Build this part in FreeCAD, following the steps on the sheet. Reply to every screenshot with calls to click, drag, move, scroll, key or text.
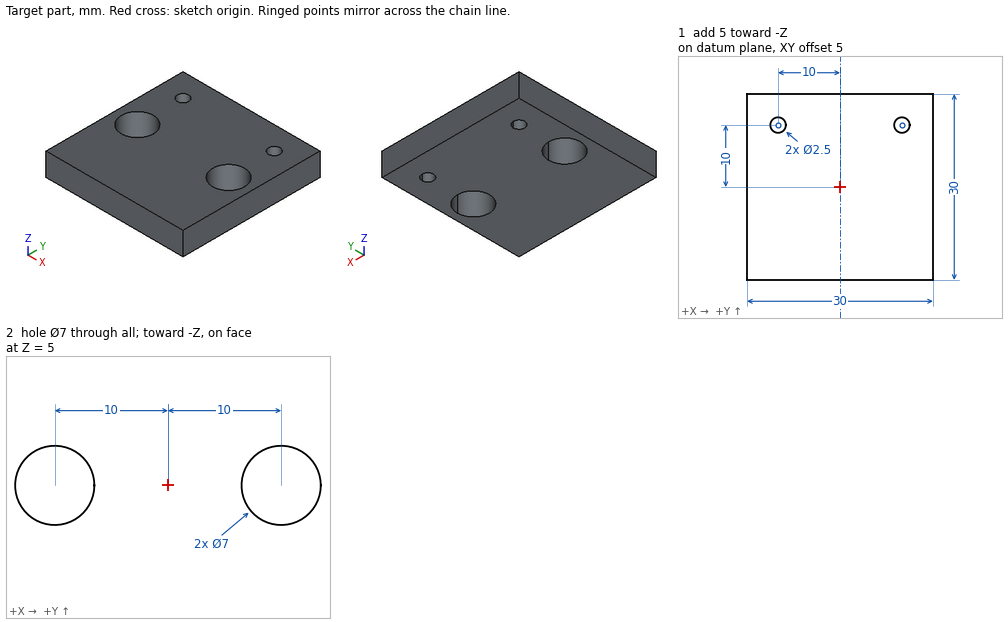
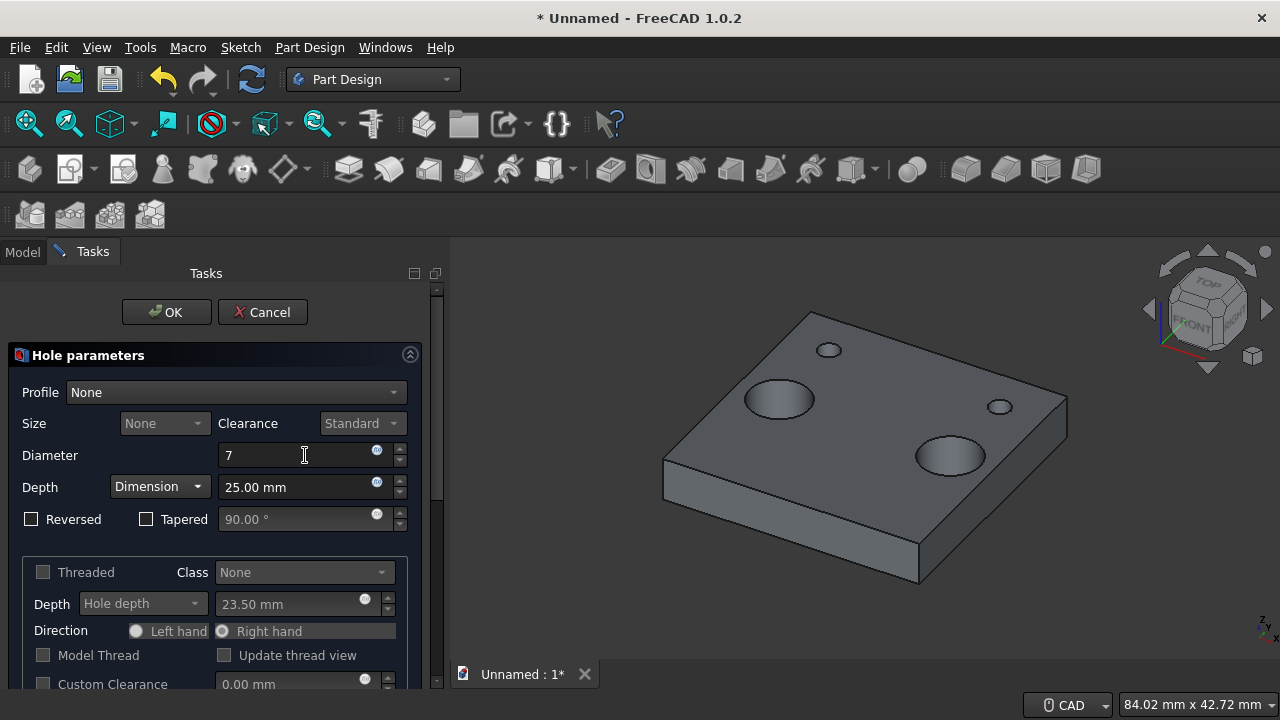
click(161, 486)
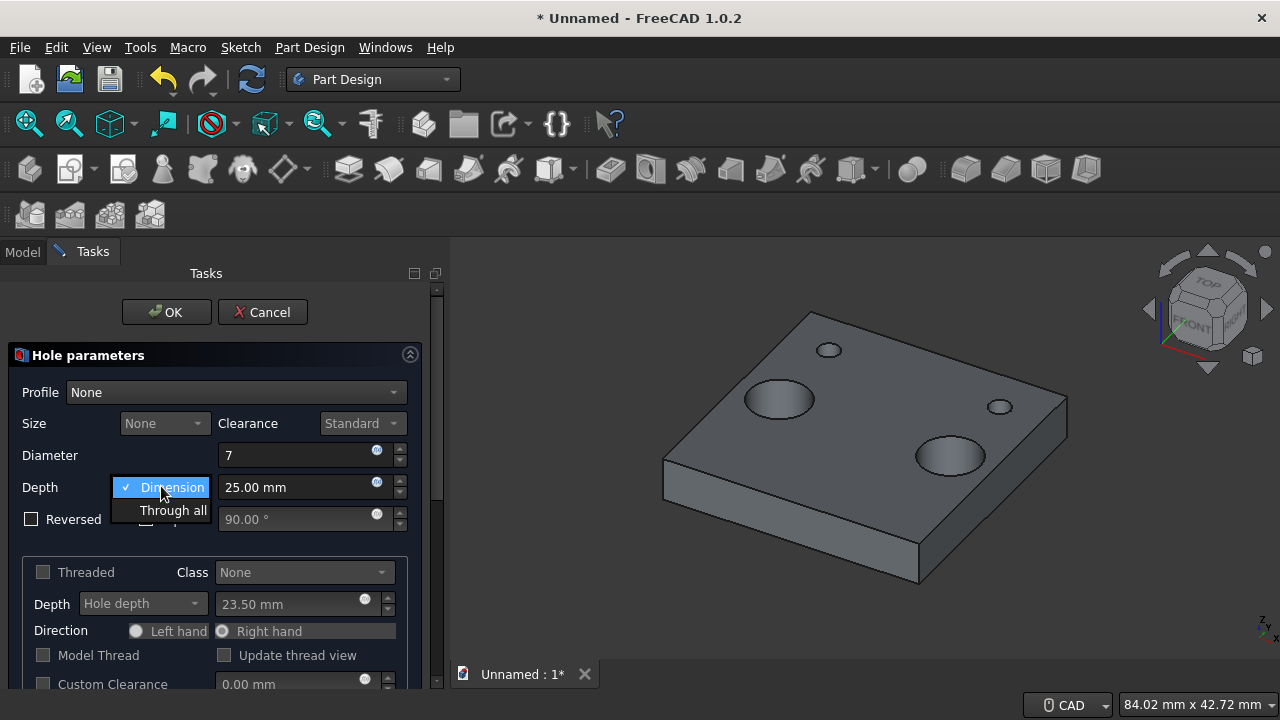
click(160, 510)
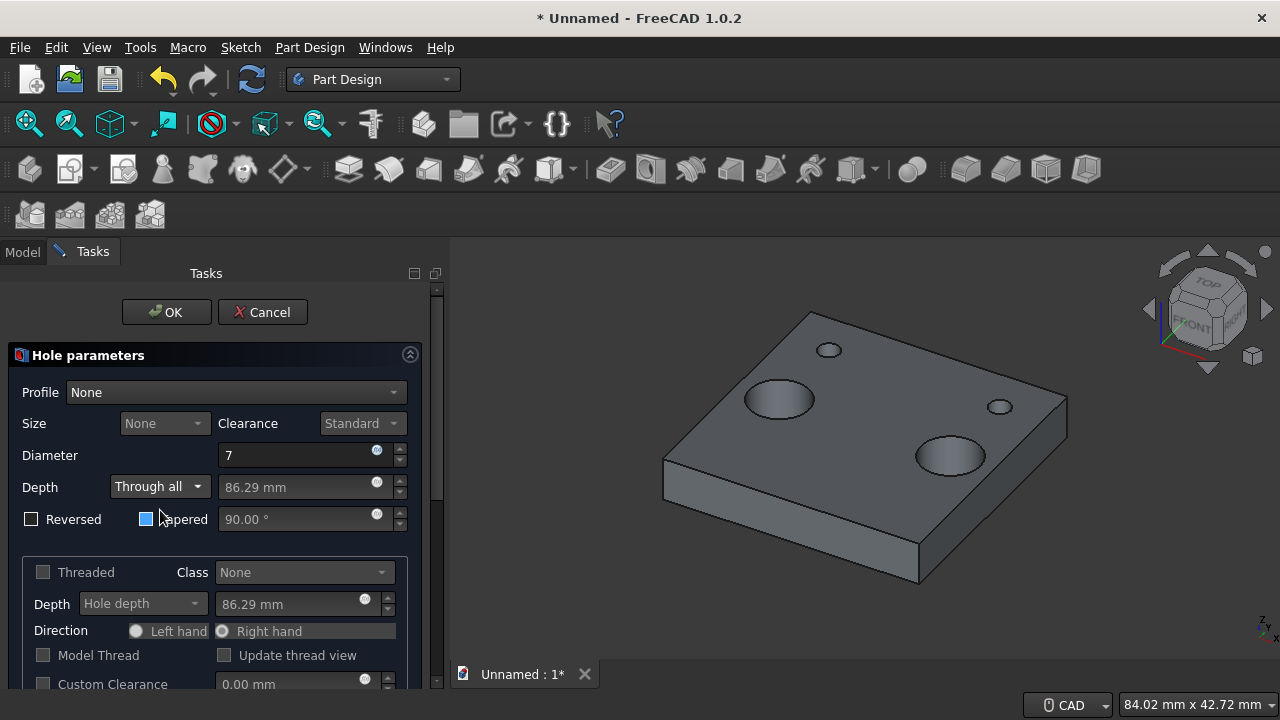
click(167, 312)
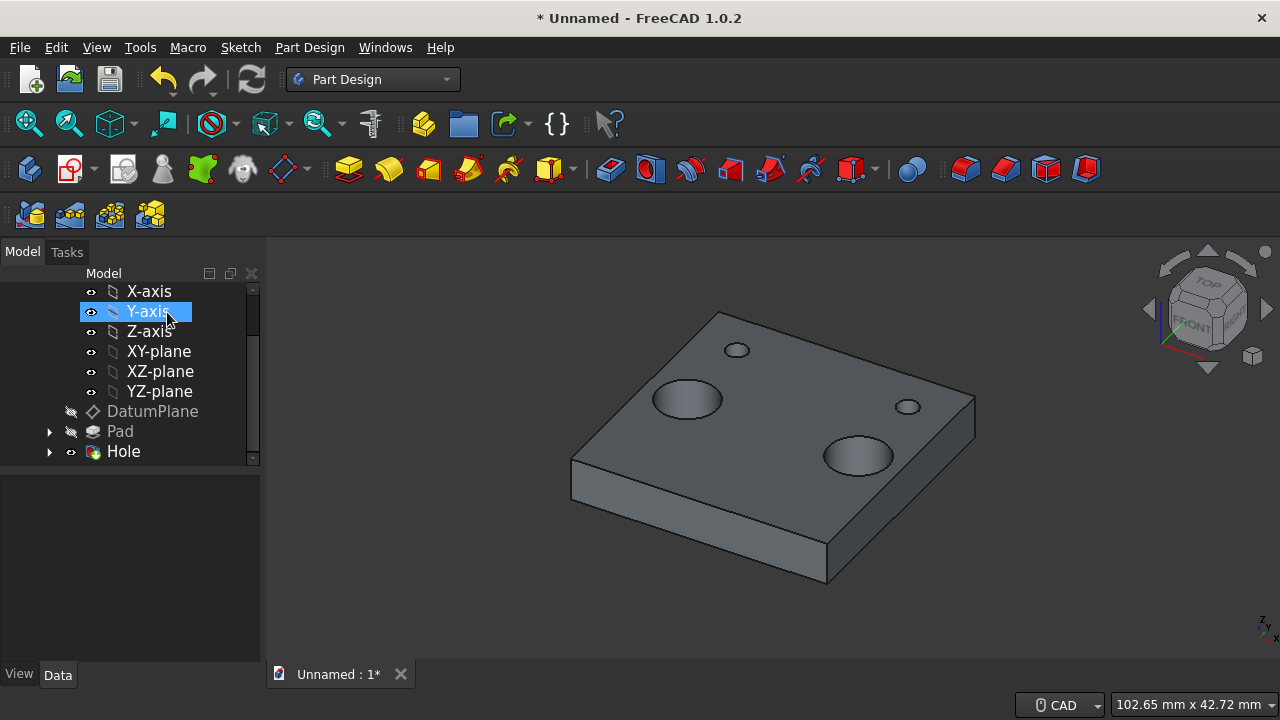
key(0)